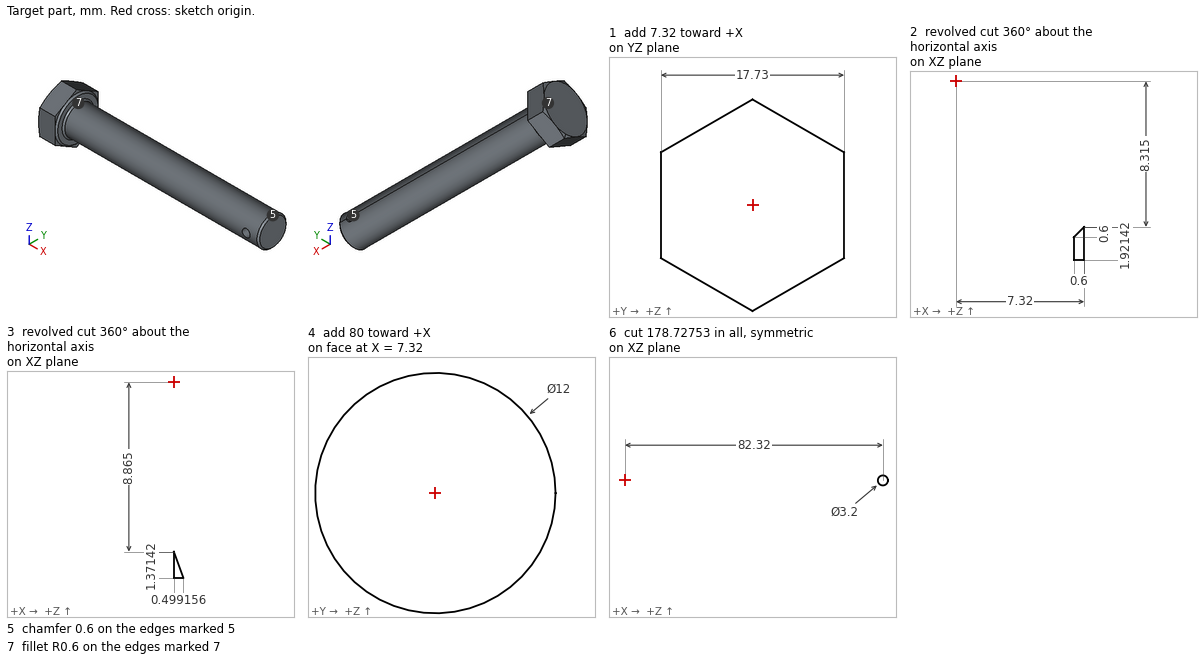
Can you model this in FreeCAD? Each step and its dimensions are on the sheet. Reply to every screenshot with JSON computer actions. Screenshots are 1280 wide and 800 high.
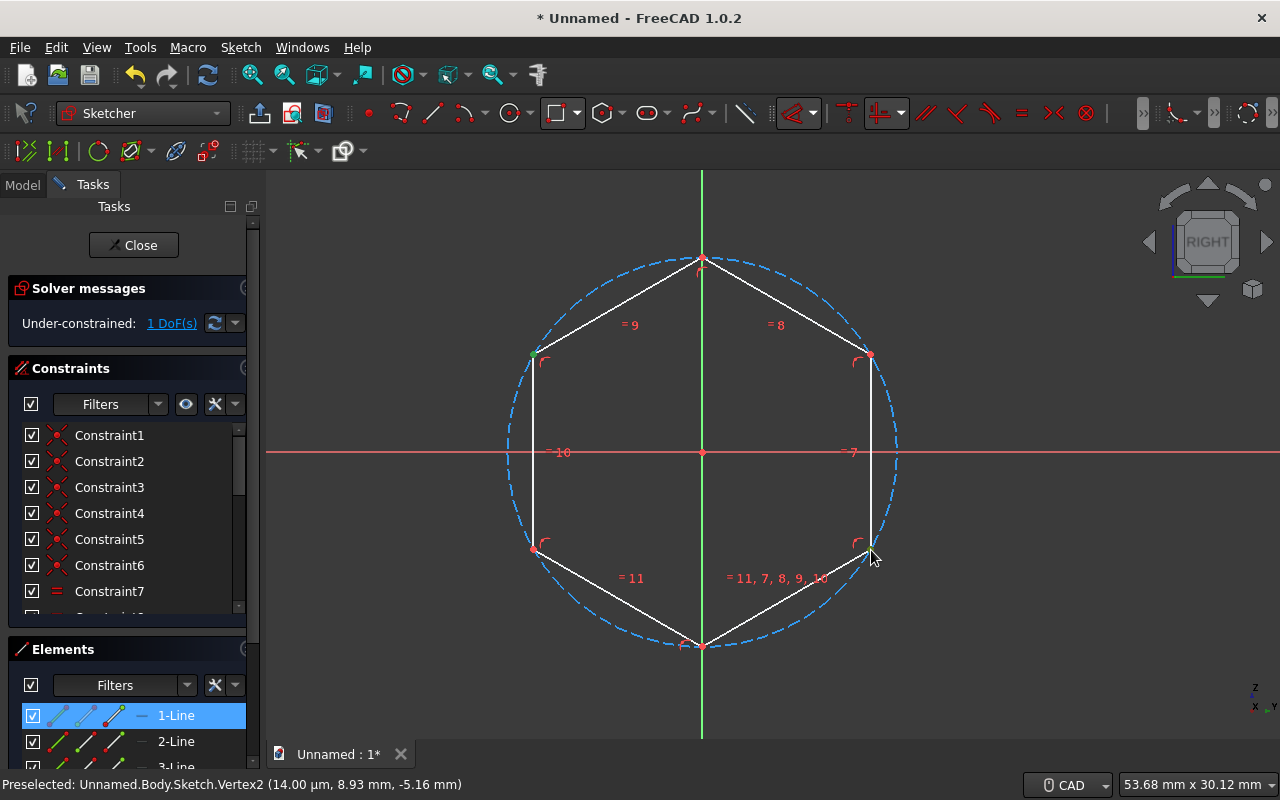
{"action": "left_click", "coordinate": [816, 114]}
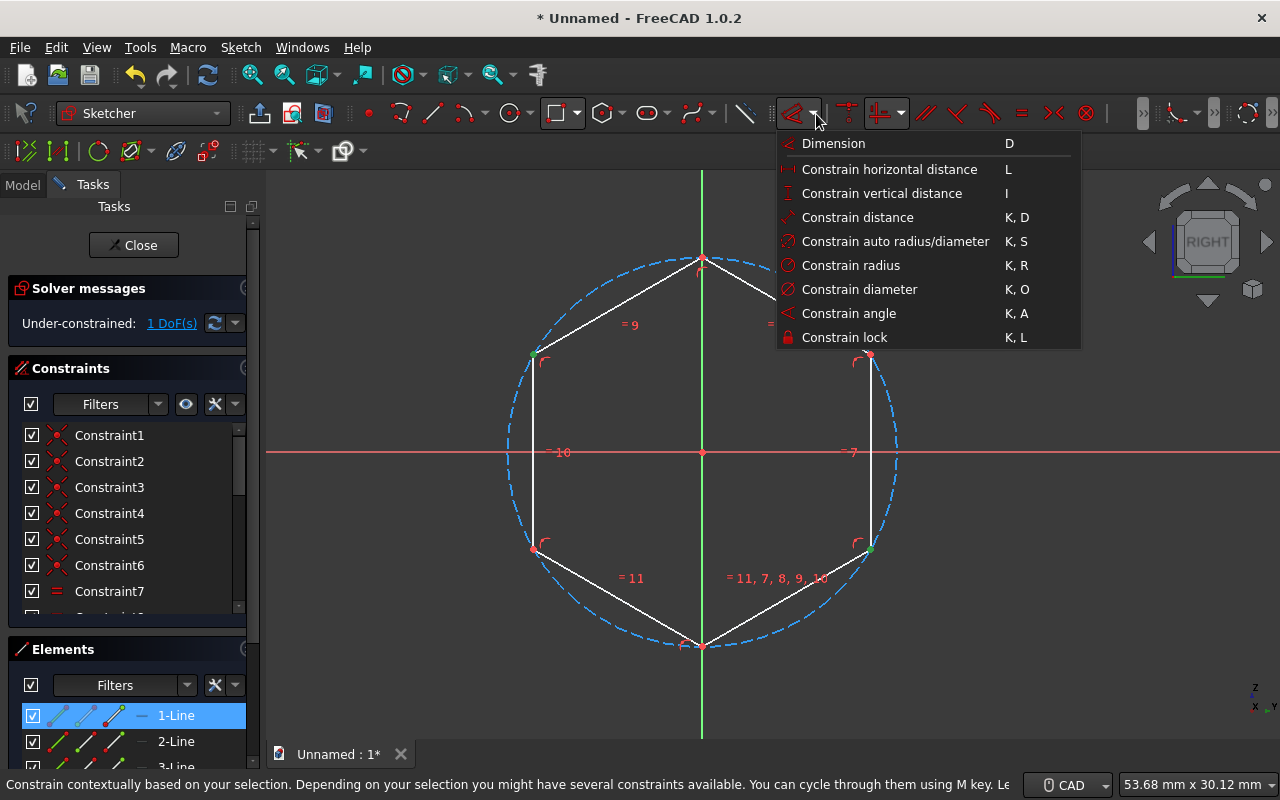
{"action": "left_click", "coordinate": [929, 169]}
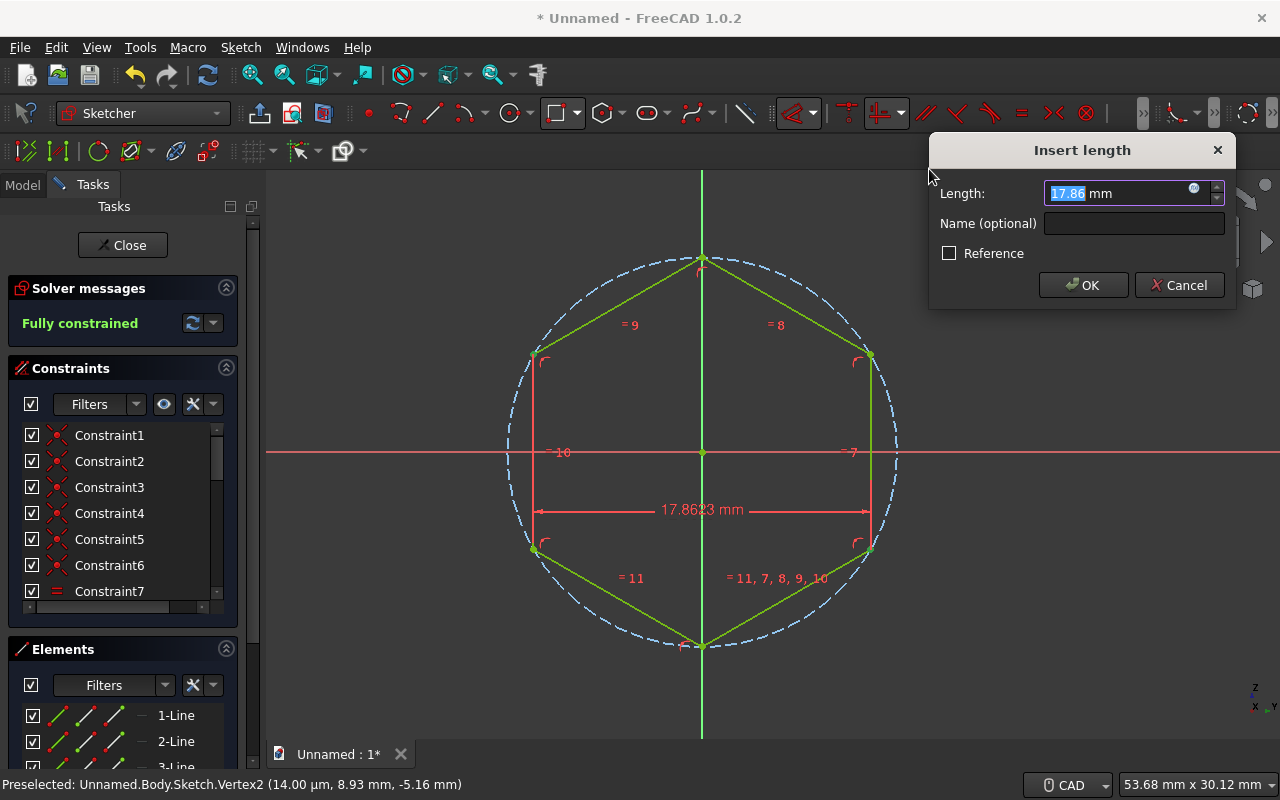
{"action": "type", "text": "17.73"}
{"action": "key", "text": "Return"}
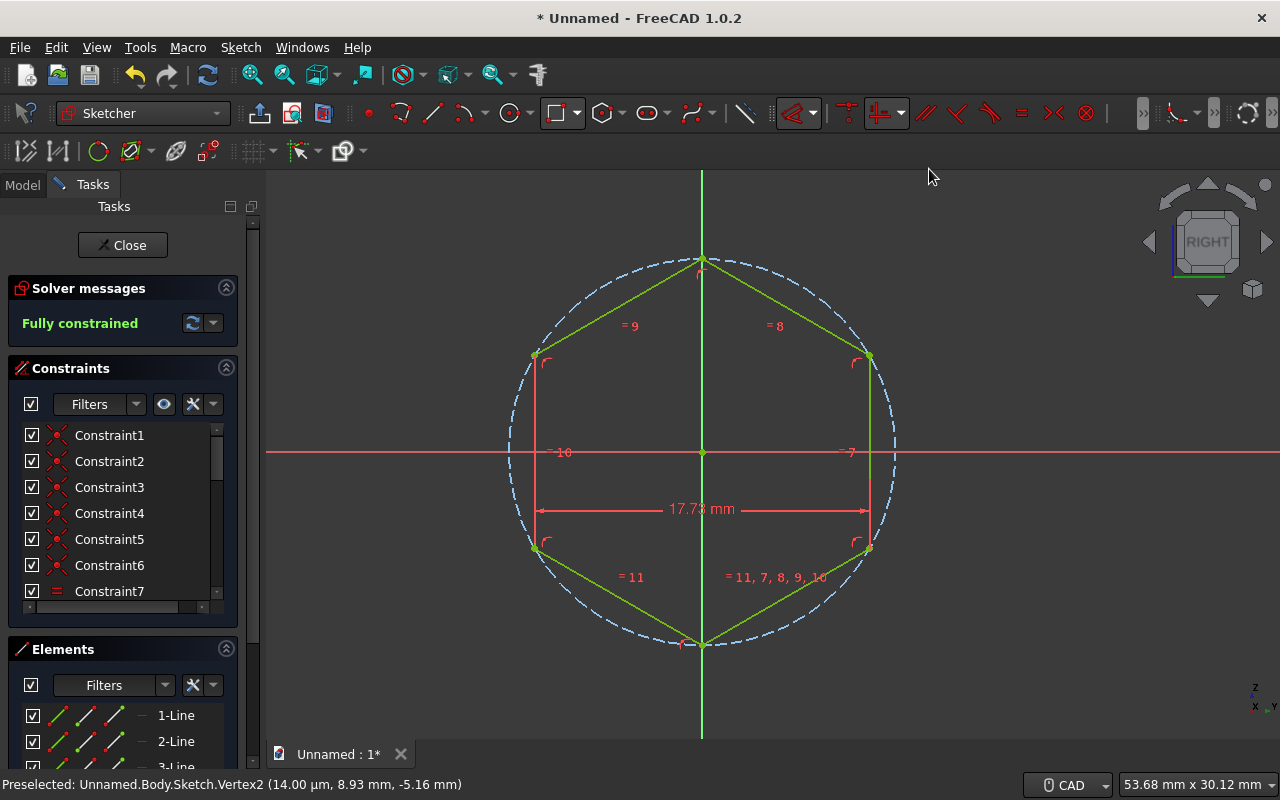
{"action": "left_click", "coordinate": [123, 245]}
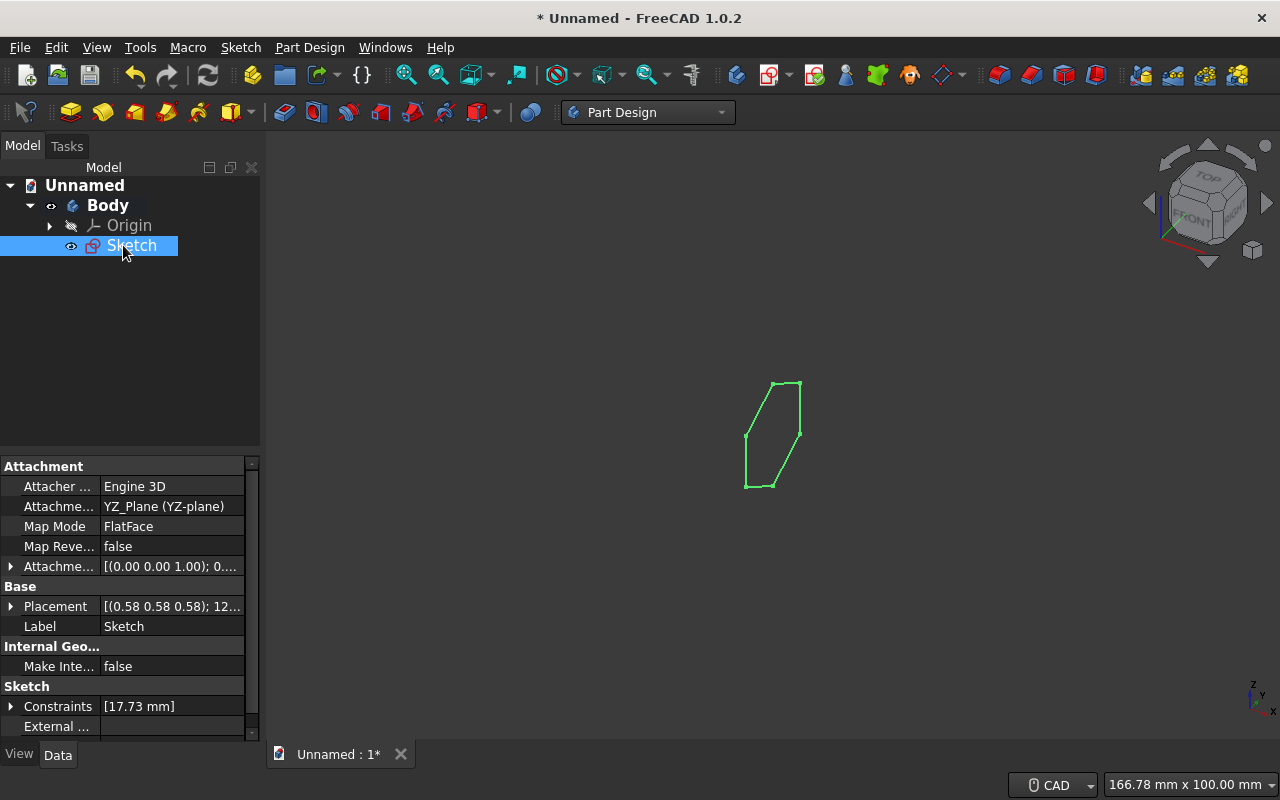
{"action": "left_click", "coordinate": [72, 112]}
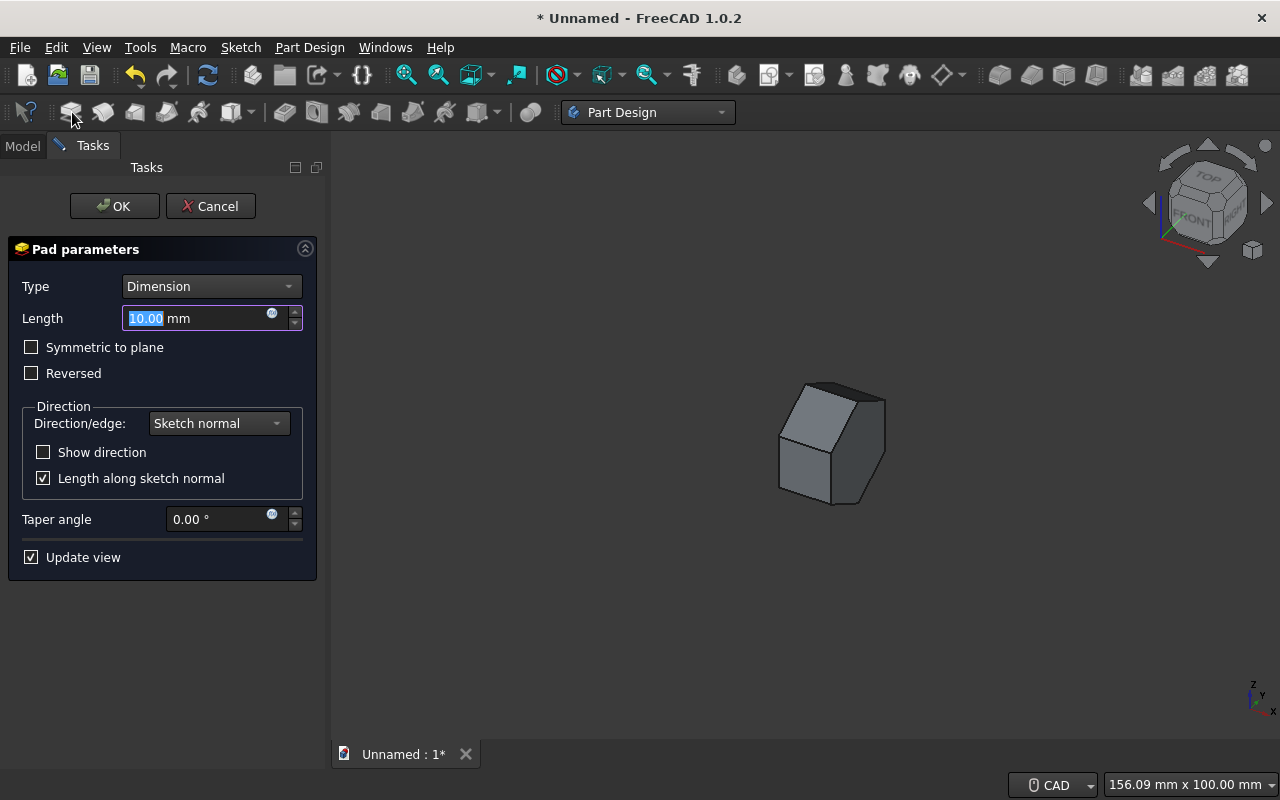
{"action": "type", "text": "7.32"}
{"action": "key", "text": "Tab"}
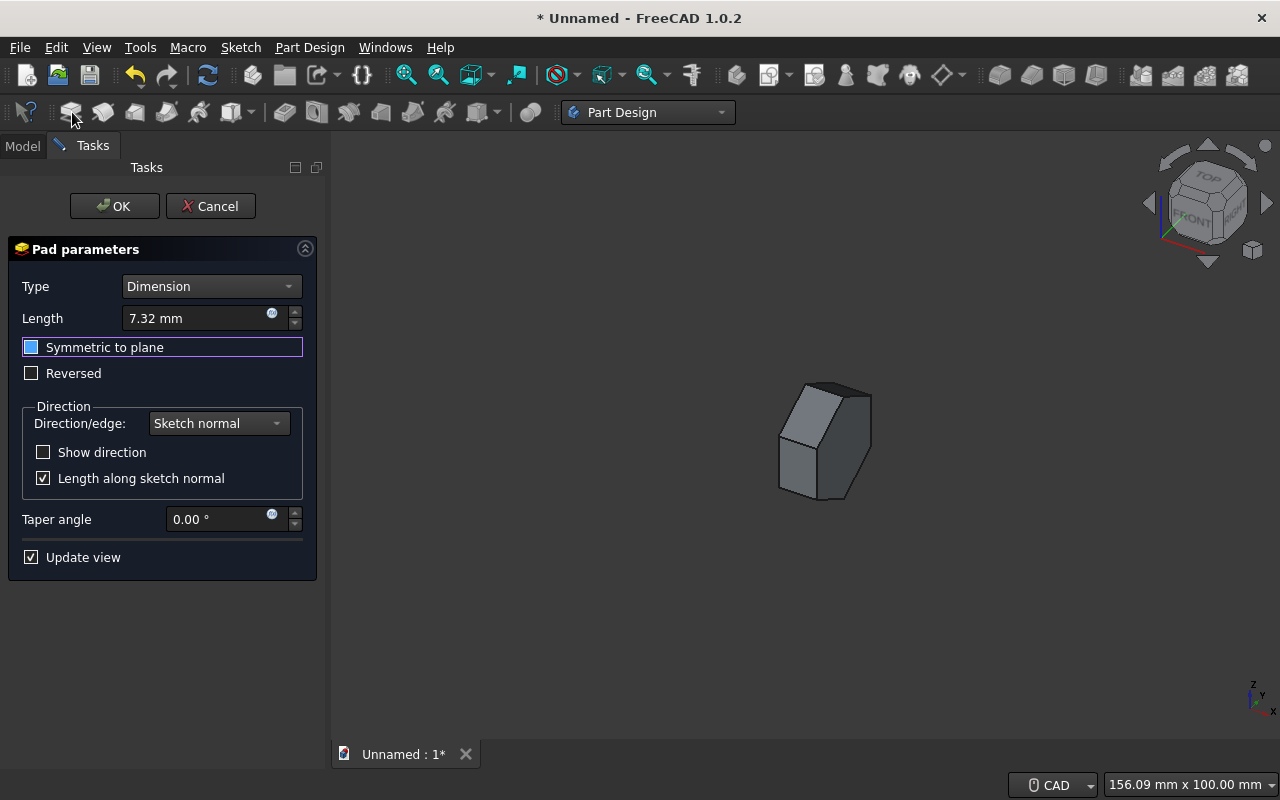
{"action": "left_click", "coordinate": [115, 206]}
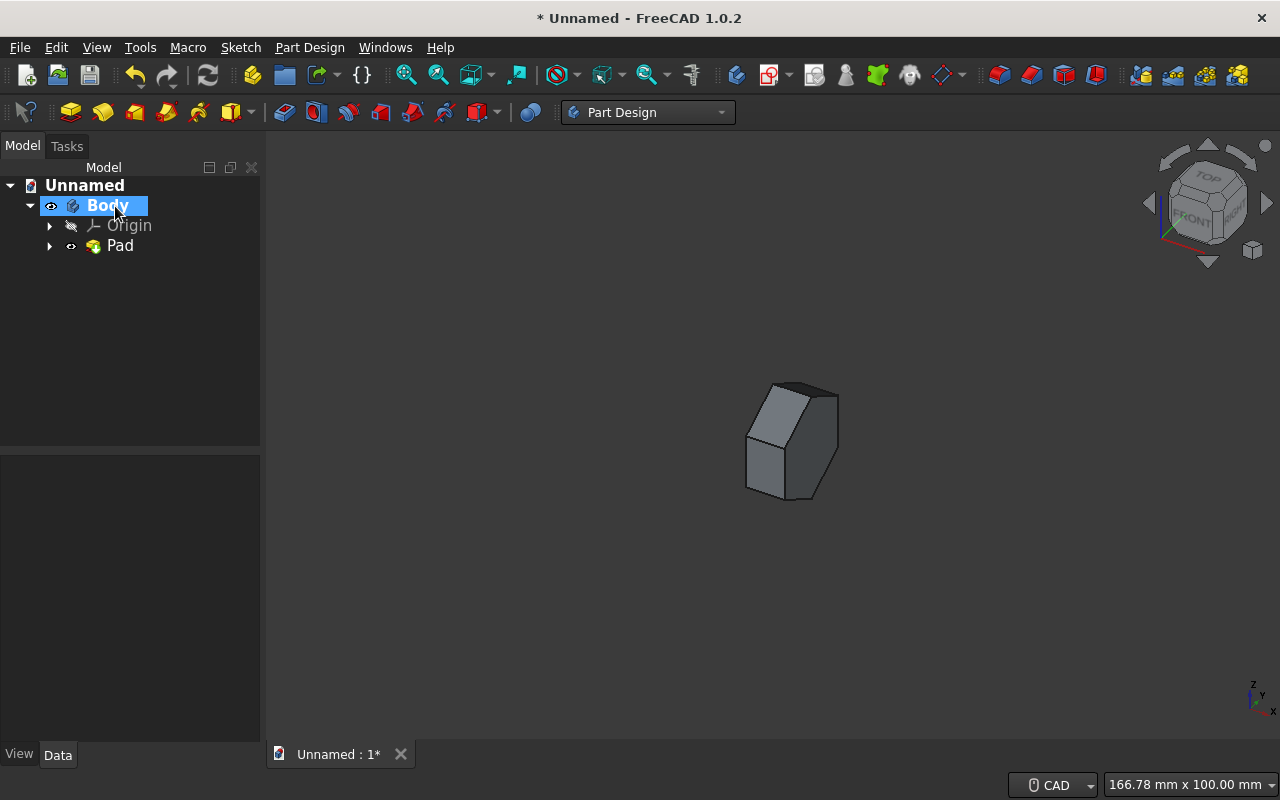
{"action": "left_click", "coordinate": [408, 76]}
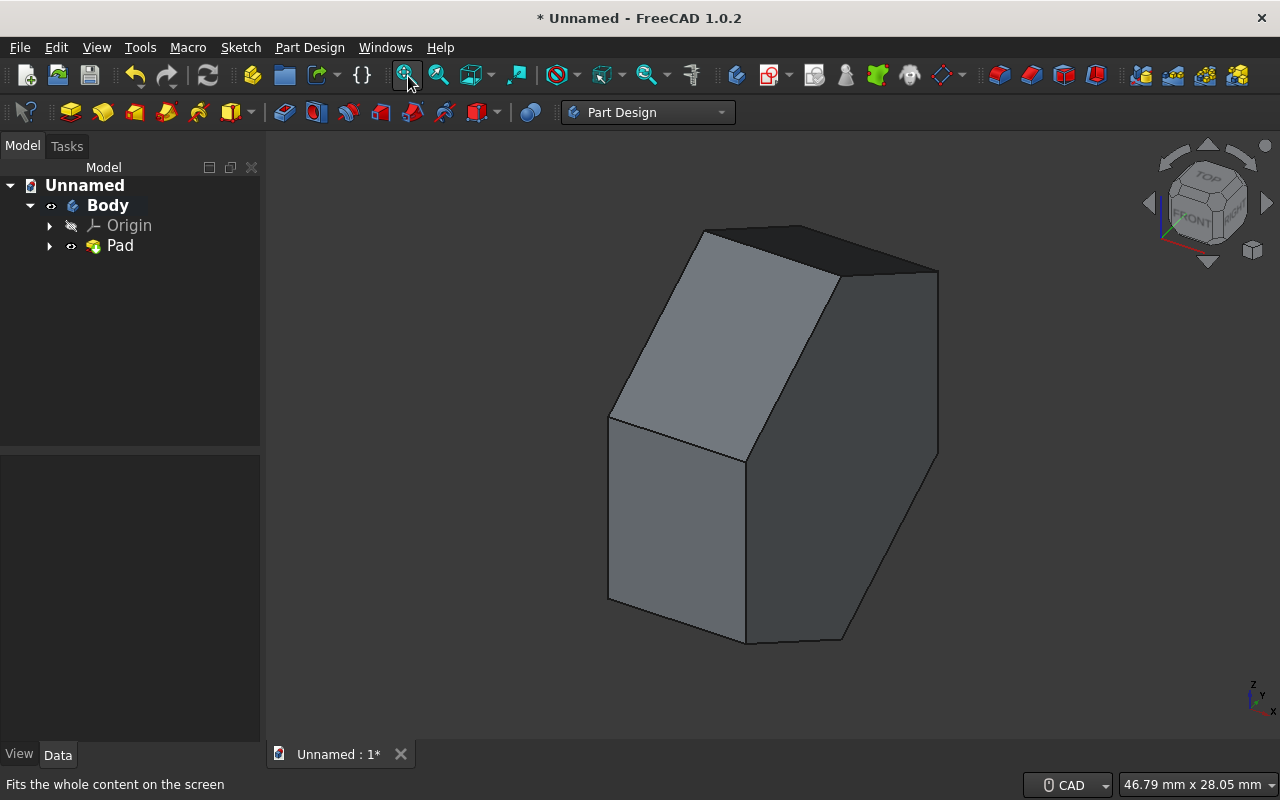
{"action": "left_click", "coordinate": [770, 76]}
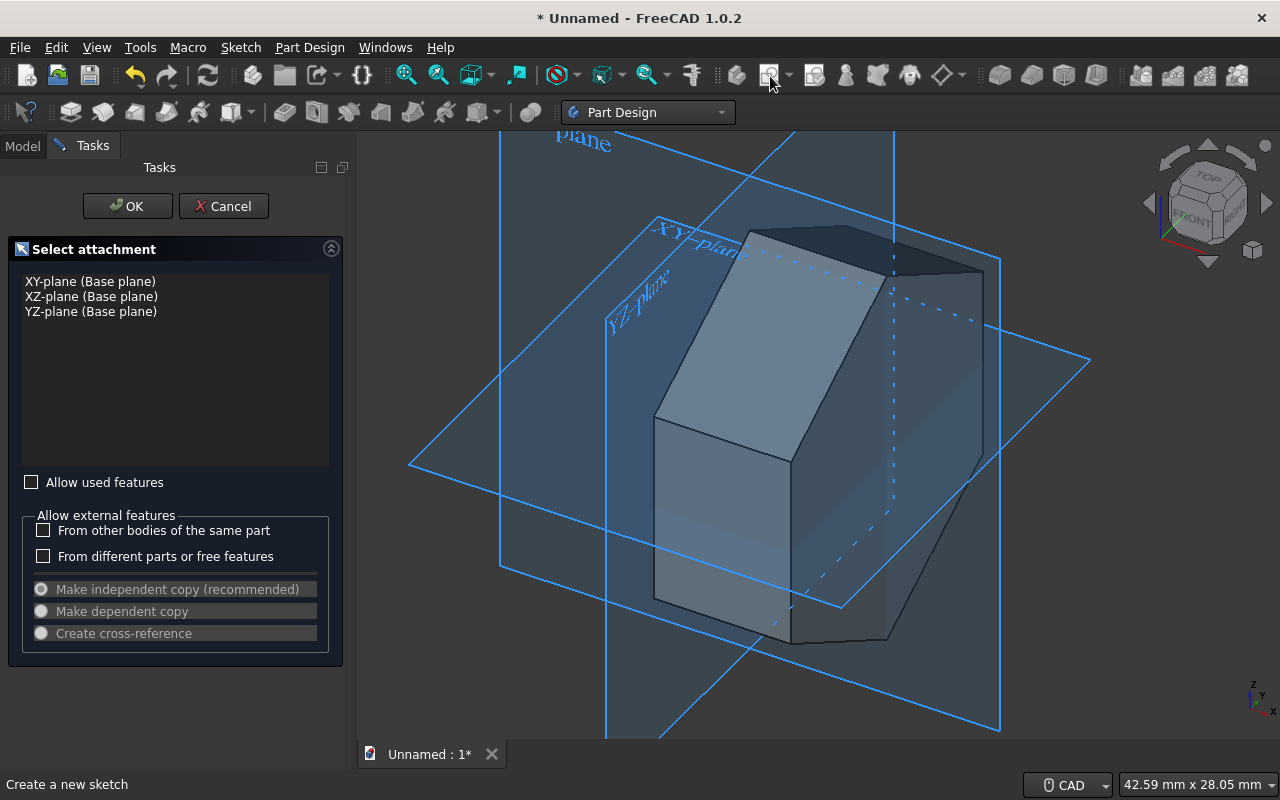
{"action": "left_click", "coordinate": [82, 296]}